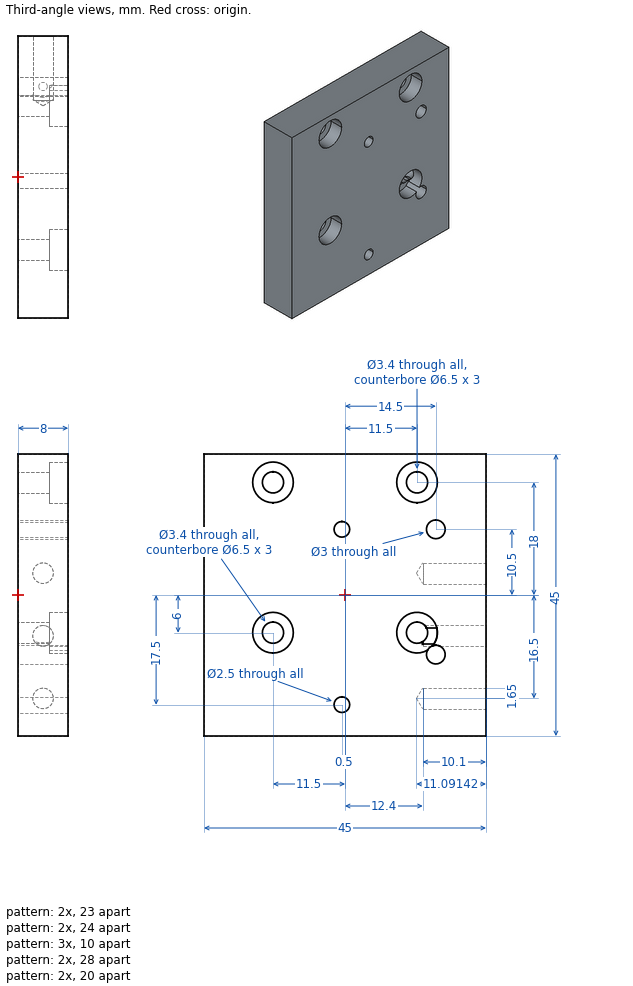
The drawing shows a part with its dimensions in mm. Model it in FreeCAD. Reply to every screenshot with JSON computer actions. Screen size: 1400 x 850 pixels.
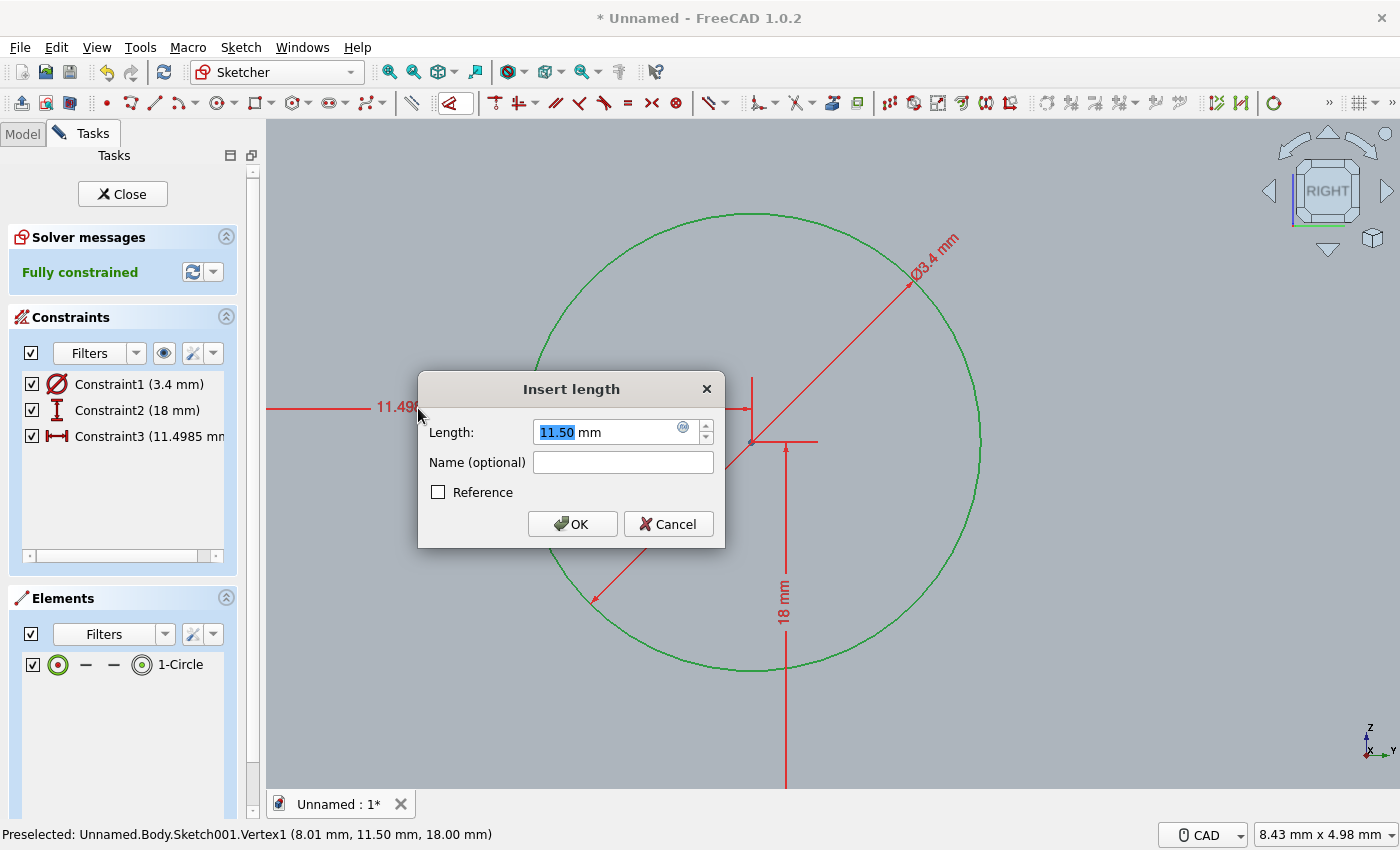
{"action": "type", "text": "11.5"}
{"action": "key", "text": "Return"}
{"action": "key", "text": "Escape"}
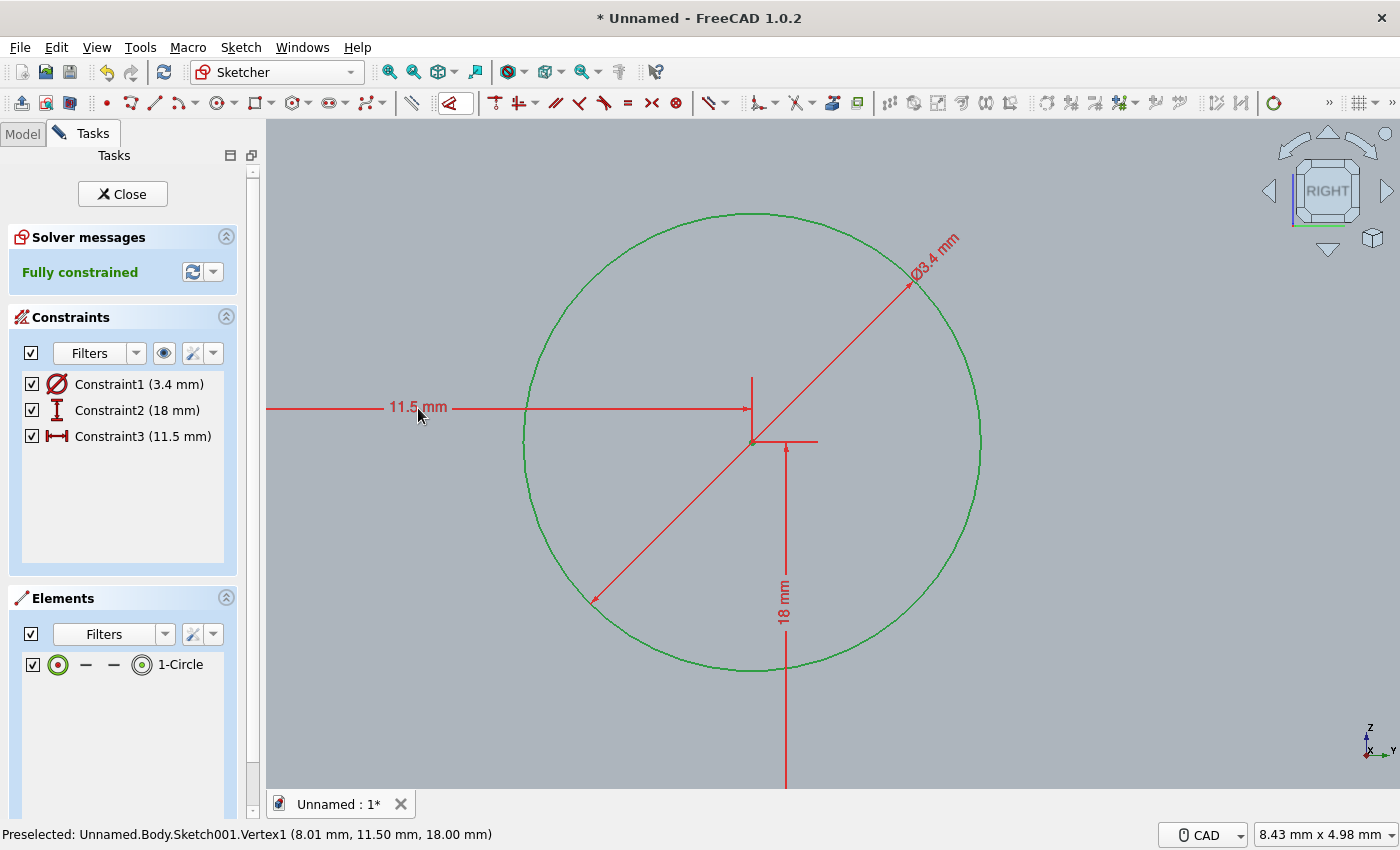
{"action": "left_click", "coordinate": [123, 194]}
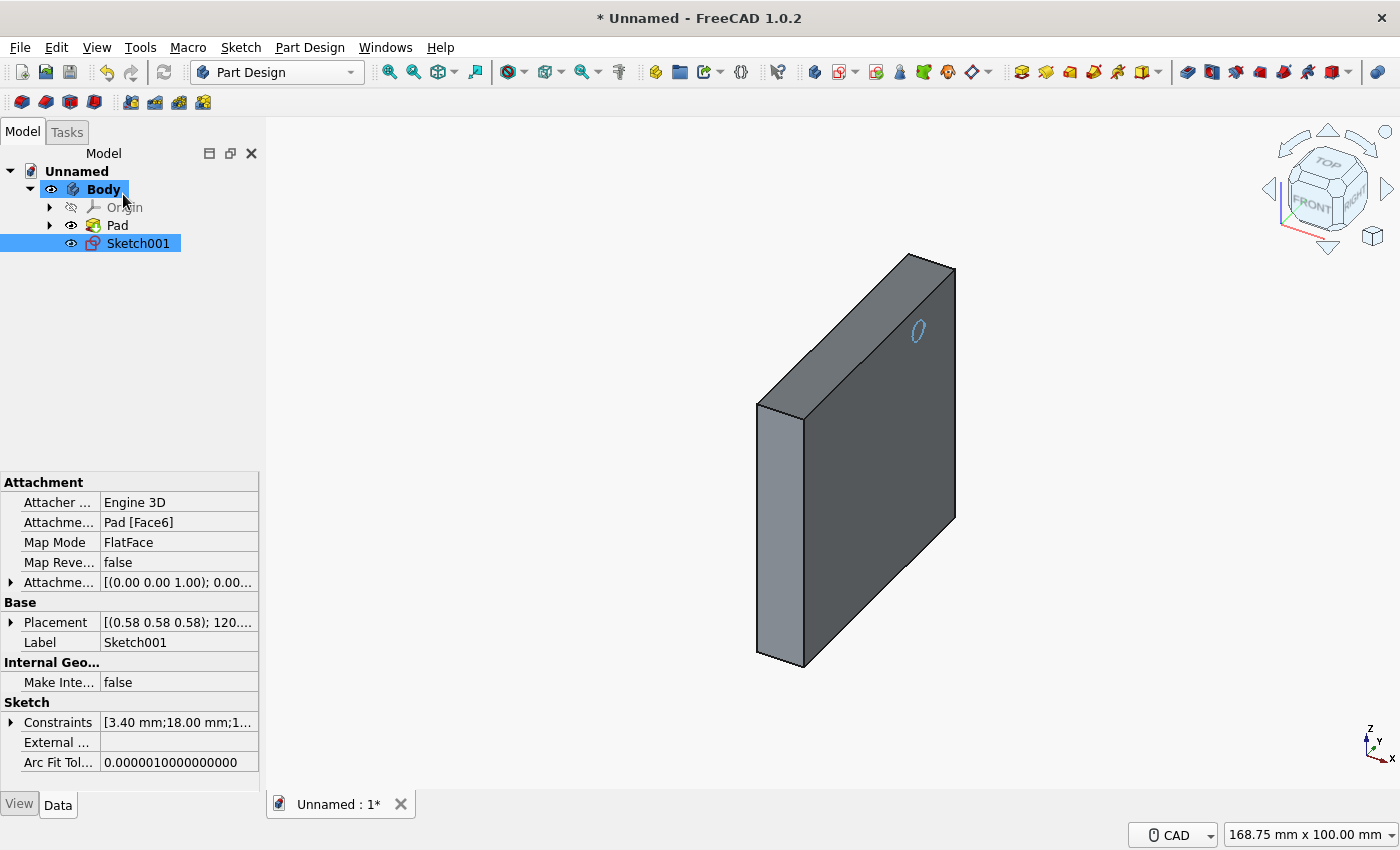
{"action": "left_click", "coordinate": [1212, 72]}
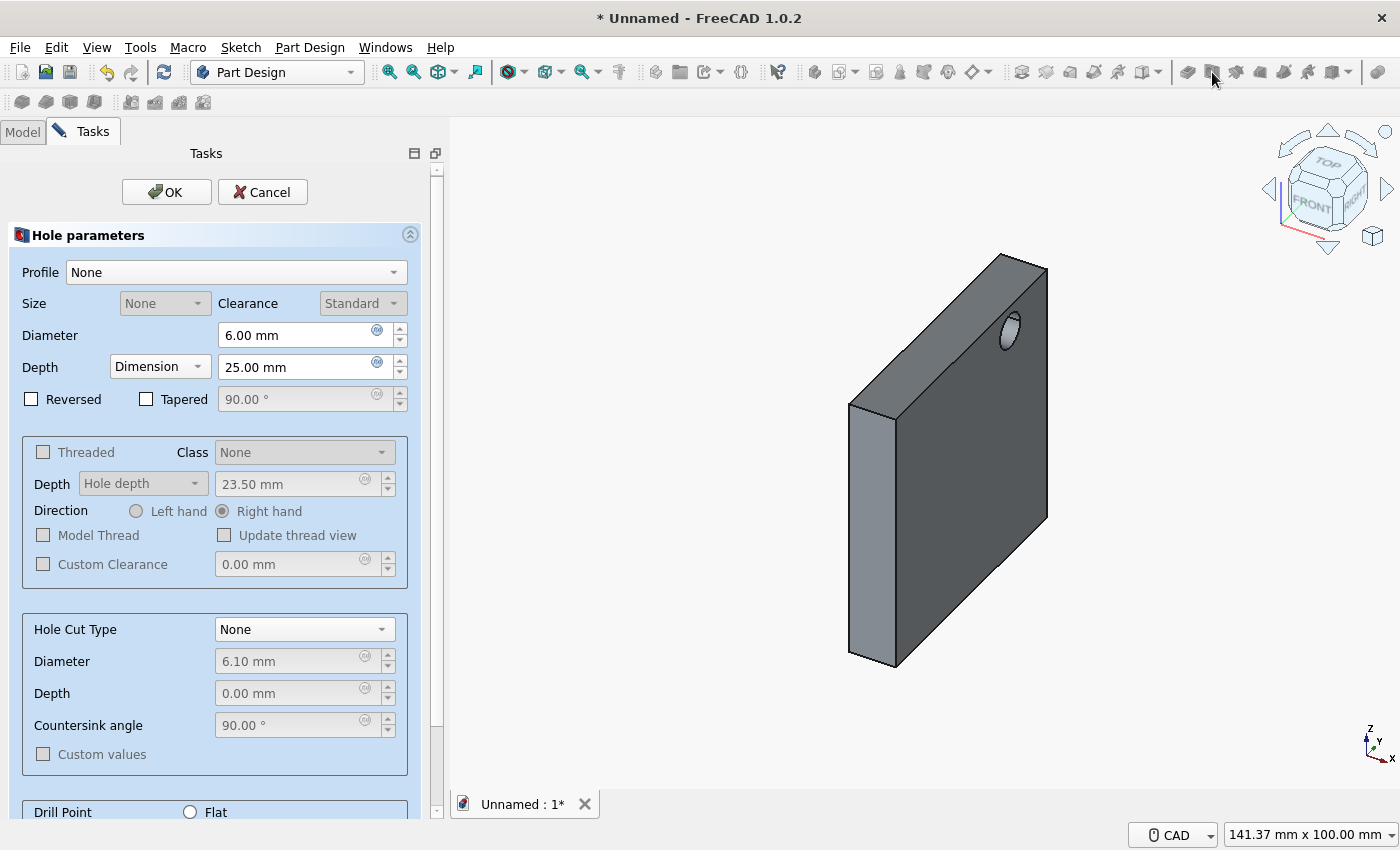
{"action": "triple_click", "coordinate": [305, 335]}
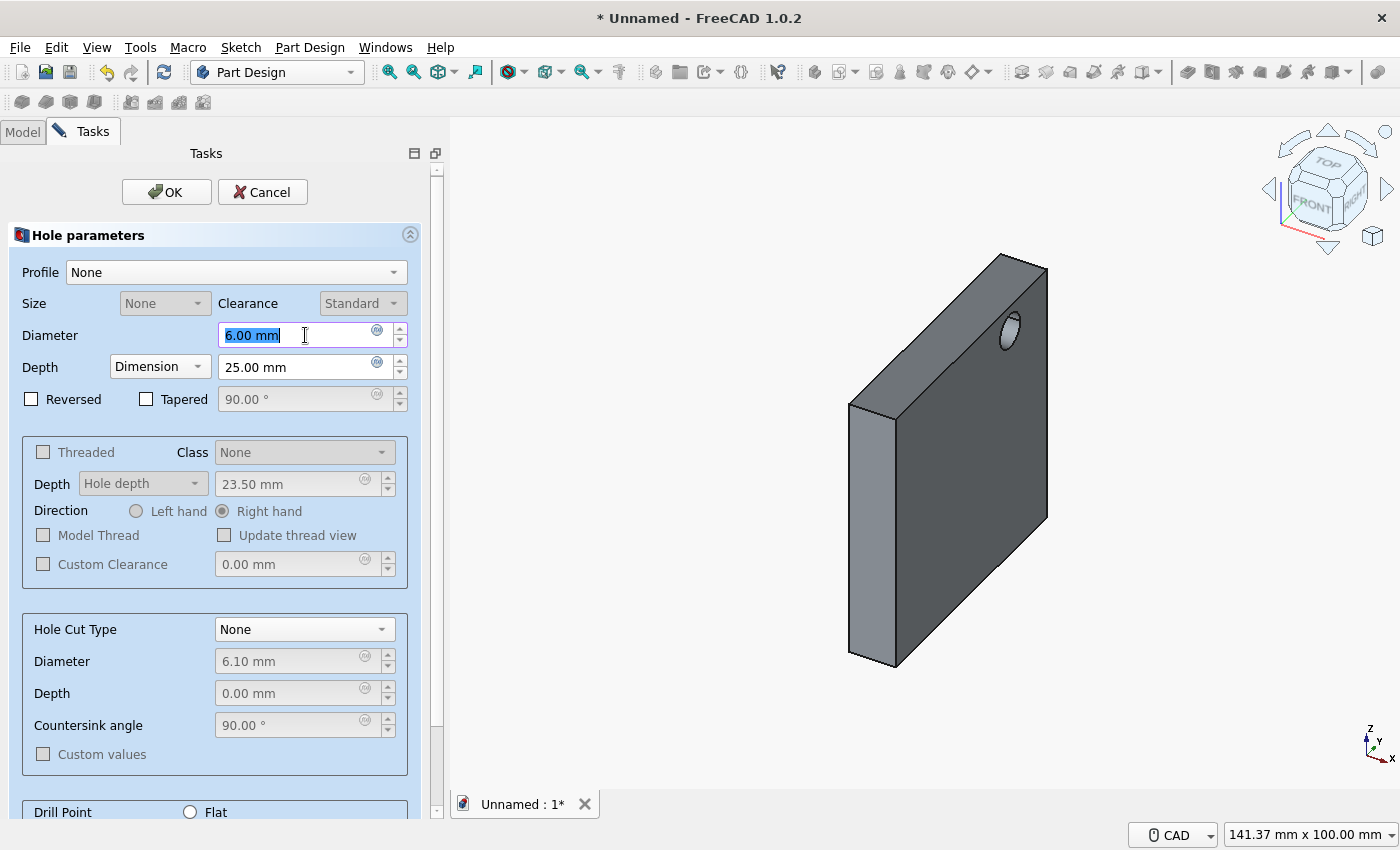
{"action": "type", "text": "3.4"}
{"action": "key", "text": "Tab"}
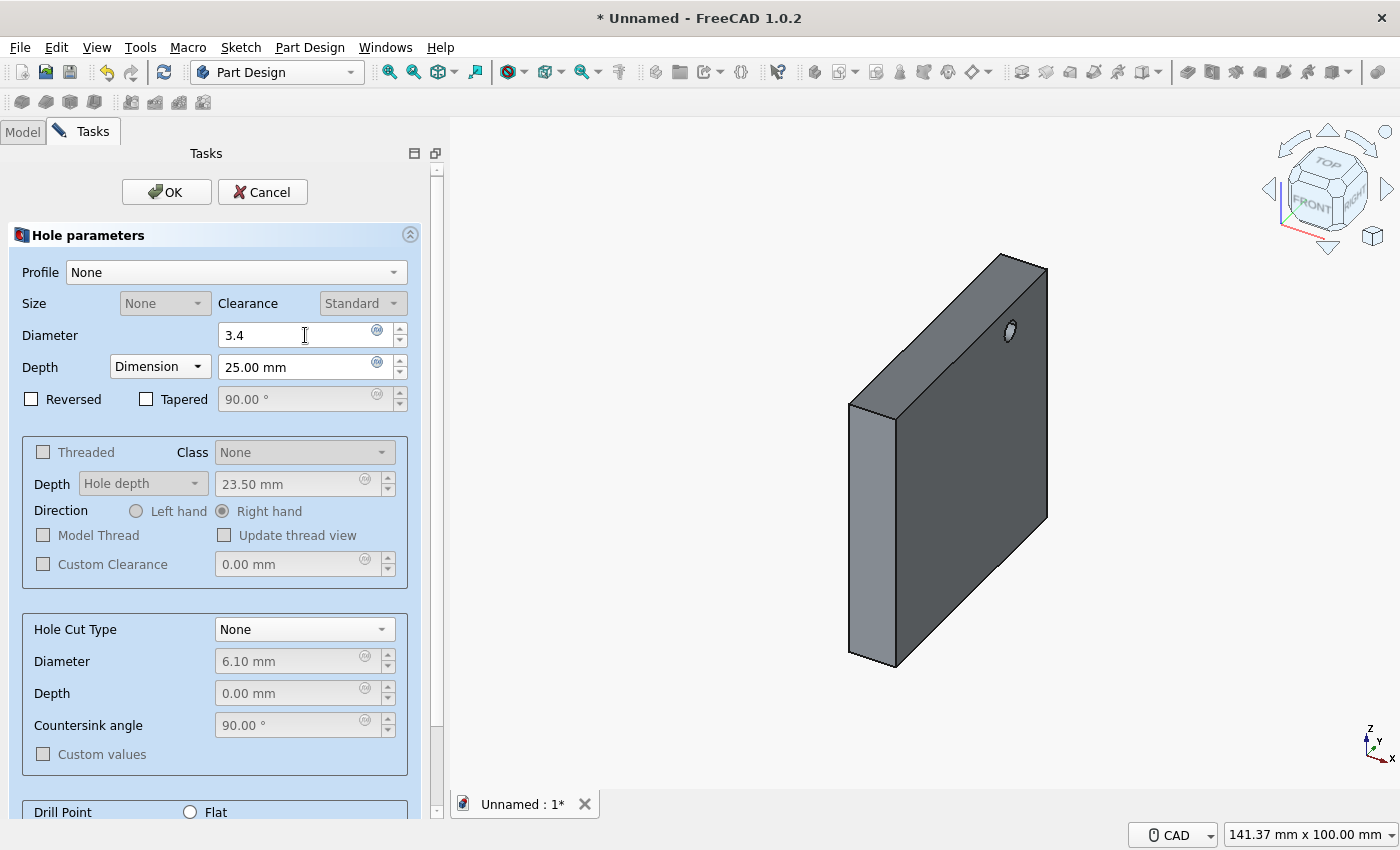
{"action": "left_click", "coordinate": [161, 366]}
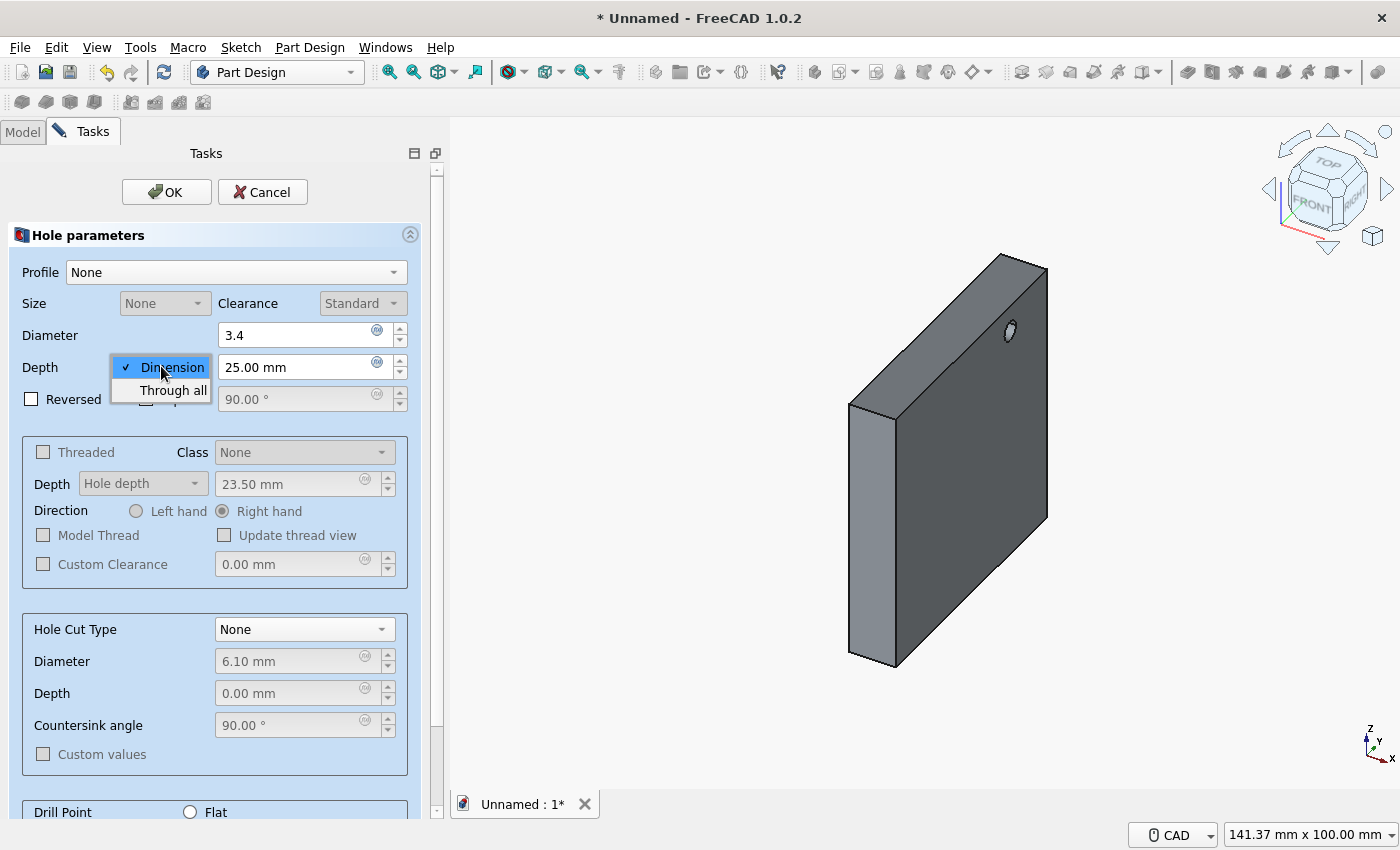
{"action": "left_click", "coordinate": [160, 390]}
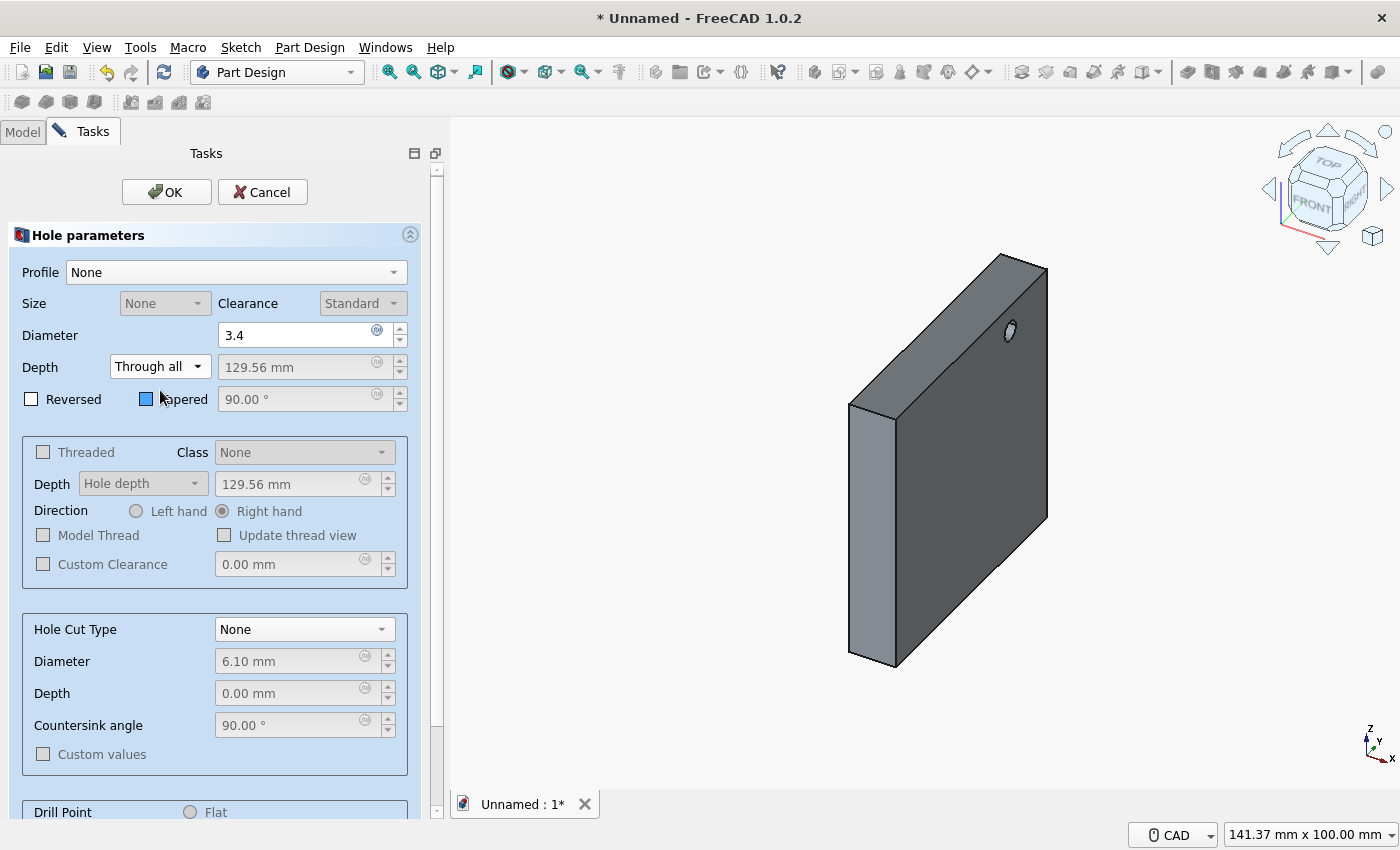
{"action": "left_click", "coordinate": [306, 630]}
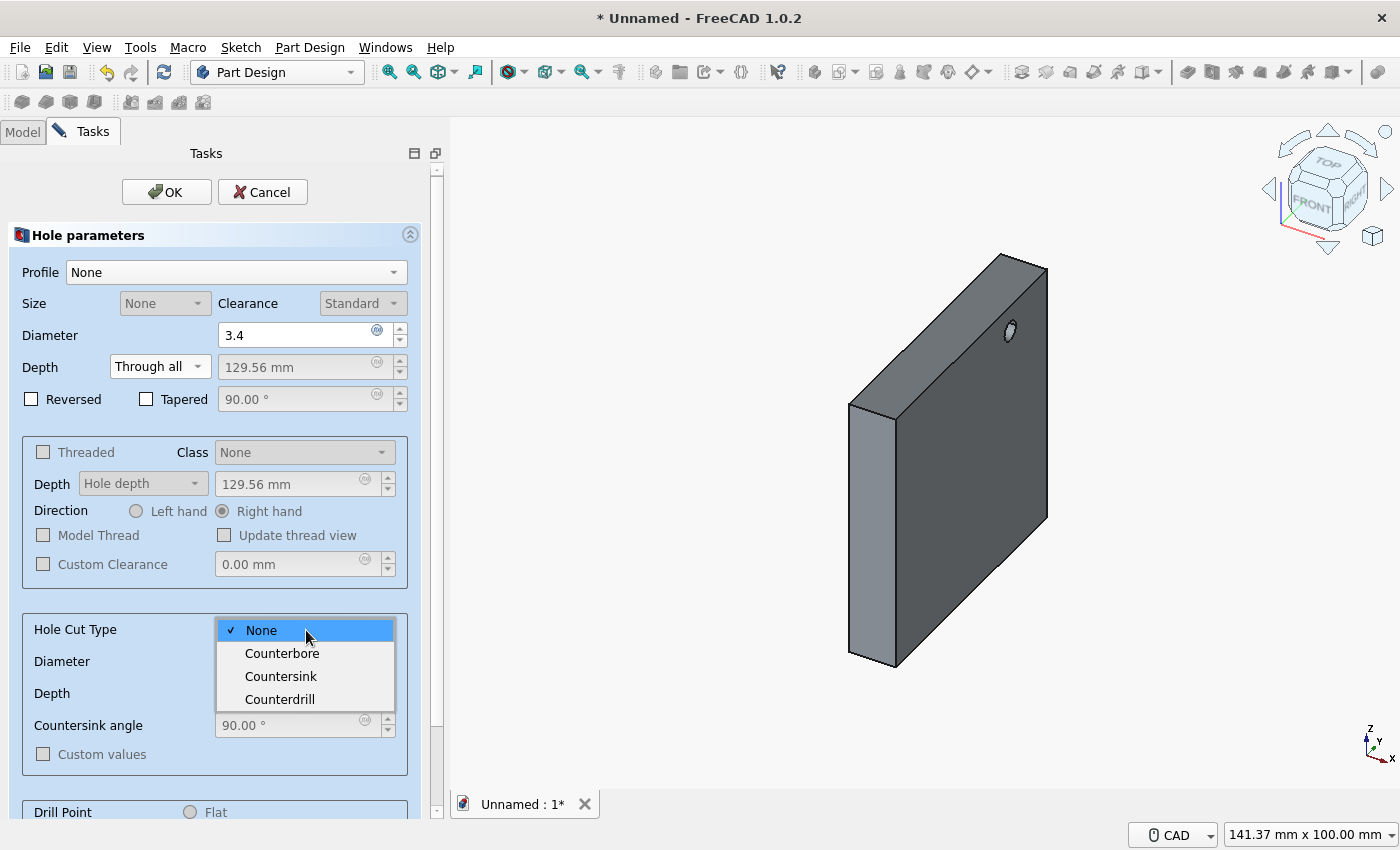
{"action": "left_click", "coordinate": [304, 654]}